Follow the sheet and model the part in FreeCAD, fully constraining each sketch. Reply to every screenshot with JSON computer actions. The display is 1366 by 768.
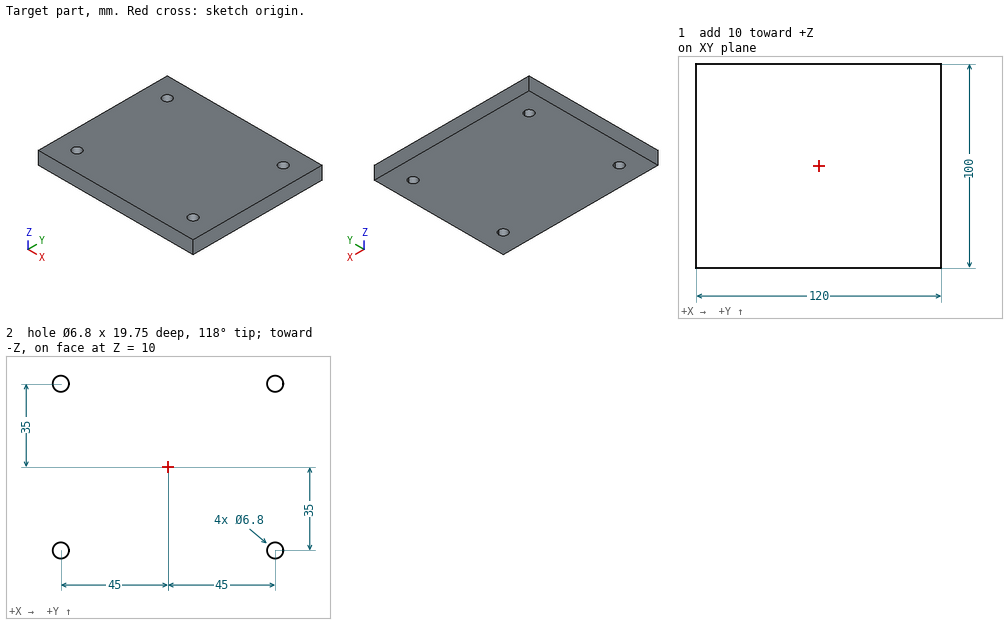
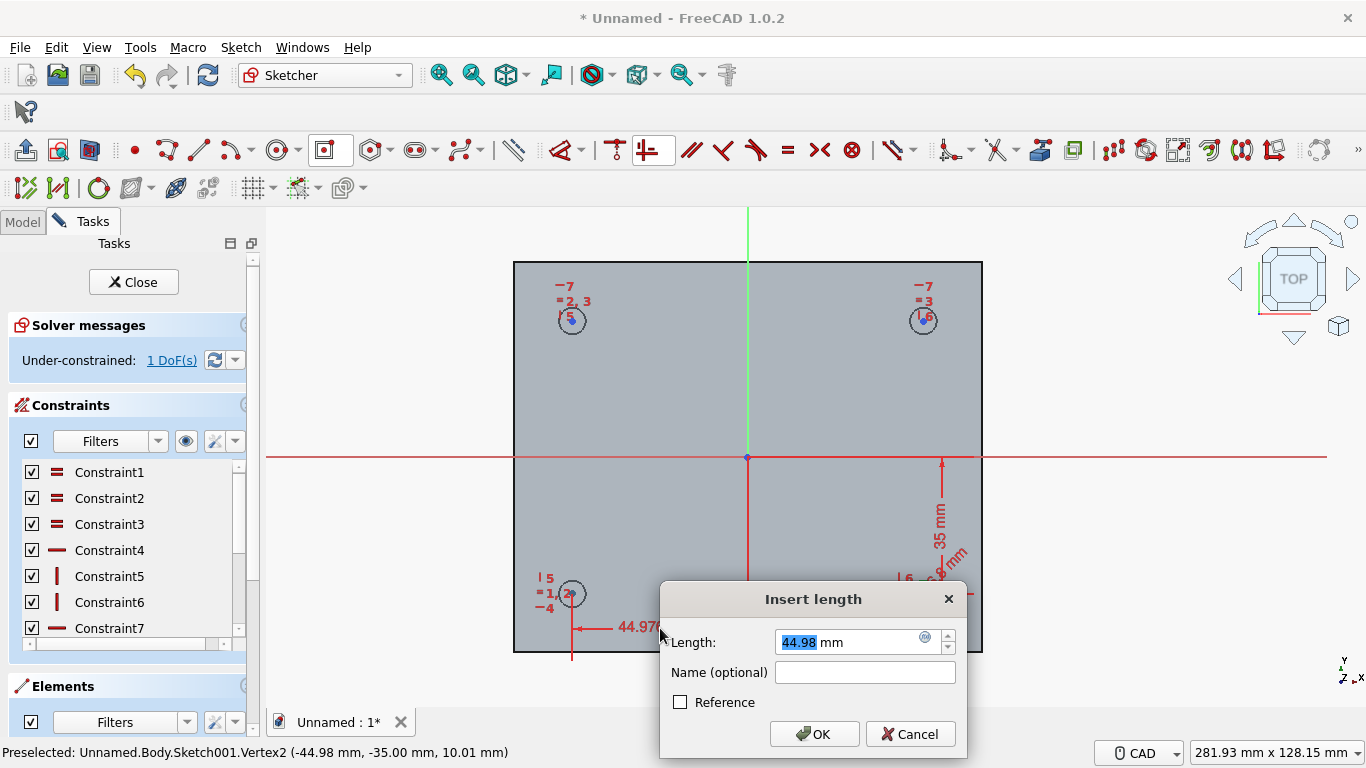
{"action": "type", "text": "45"}
{"action": "key", "text": "Return"}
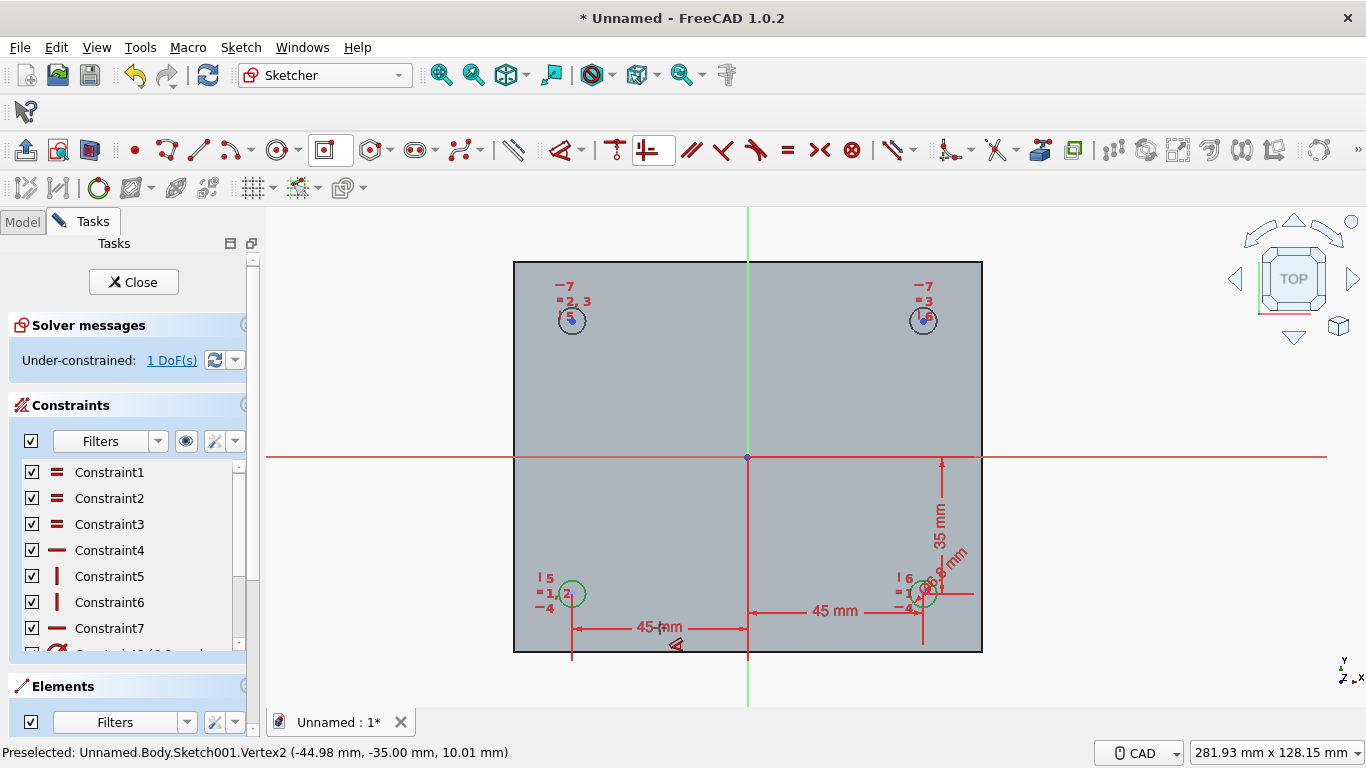
{"action": "left_click", "coordinate": [572, 321]}
{"action": "left_click", "coordinate": [538, 389]}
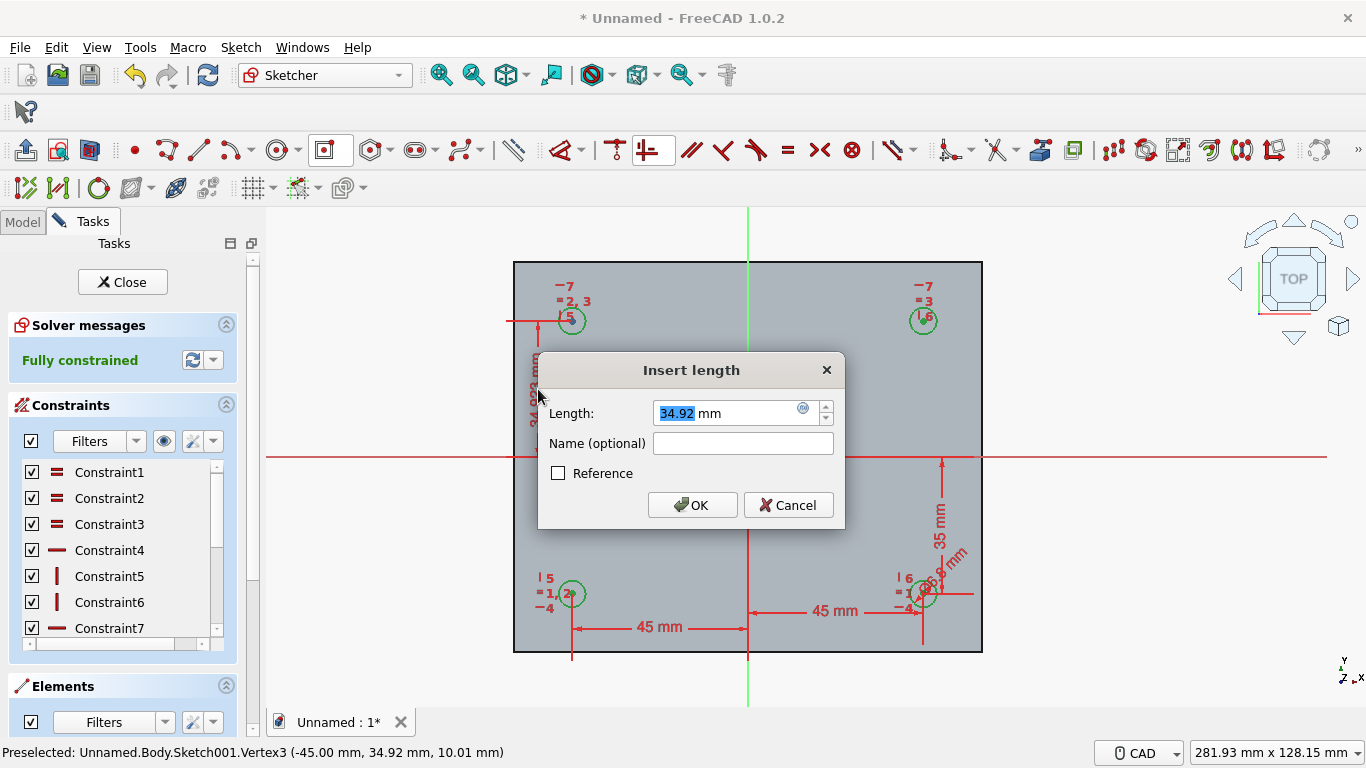
{"action": "type", "text": "35"}
{"action": "key", "text": "Return"}
{"action": "key", "text": "Escape"}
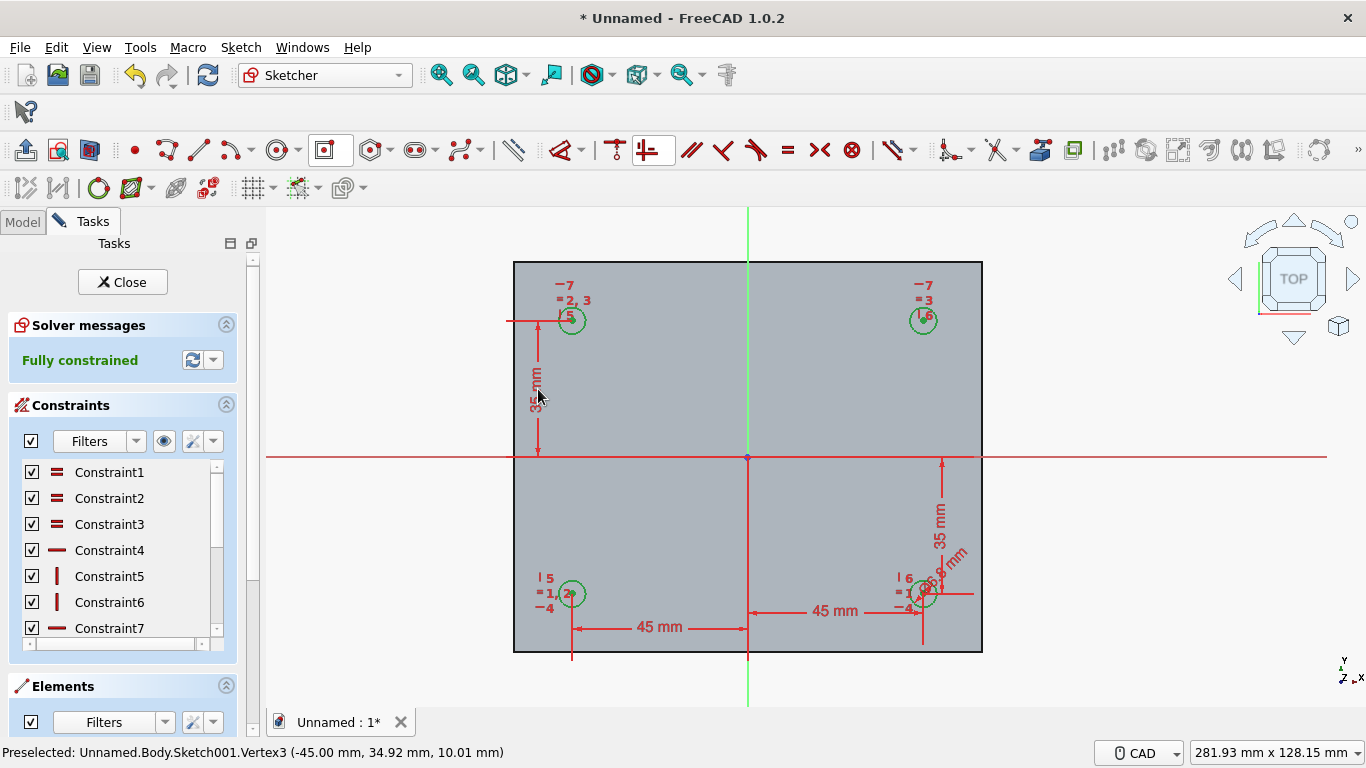
{"action": "left_click", "coordinate": [123, 282]}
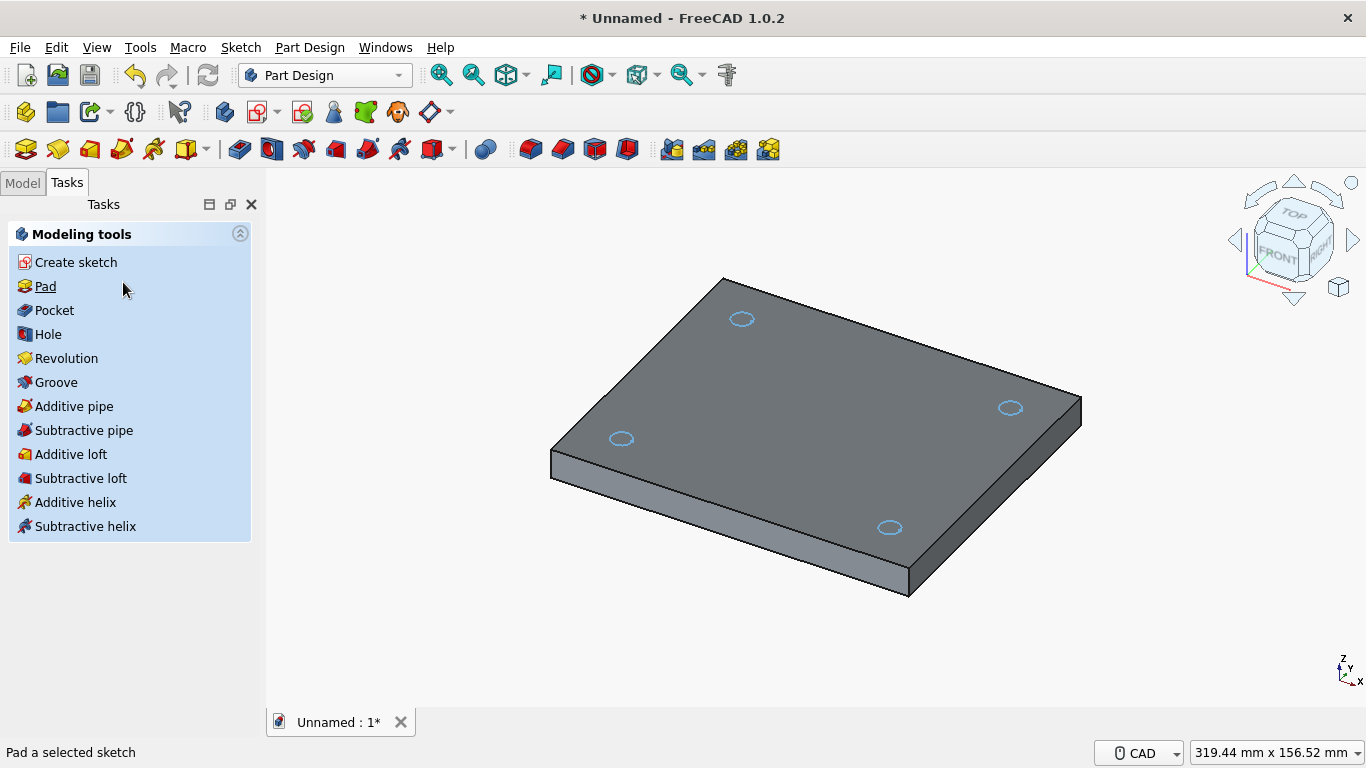
{"action": "left_click", "coordinate": [272, 150]}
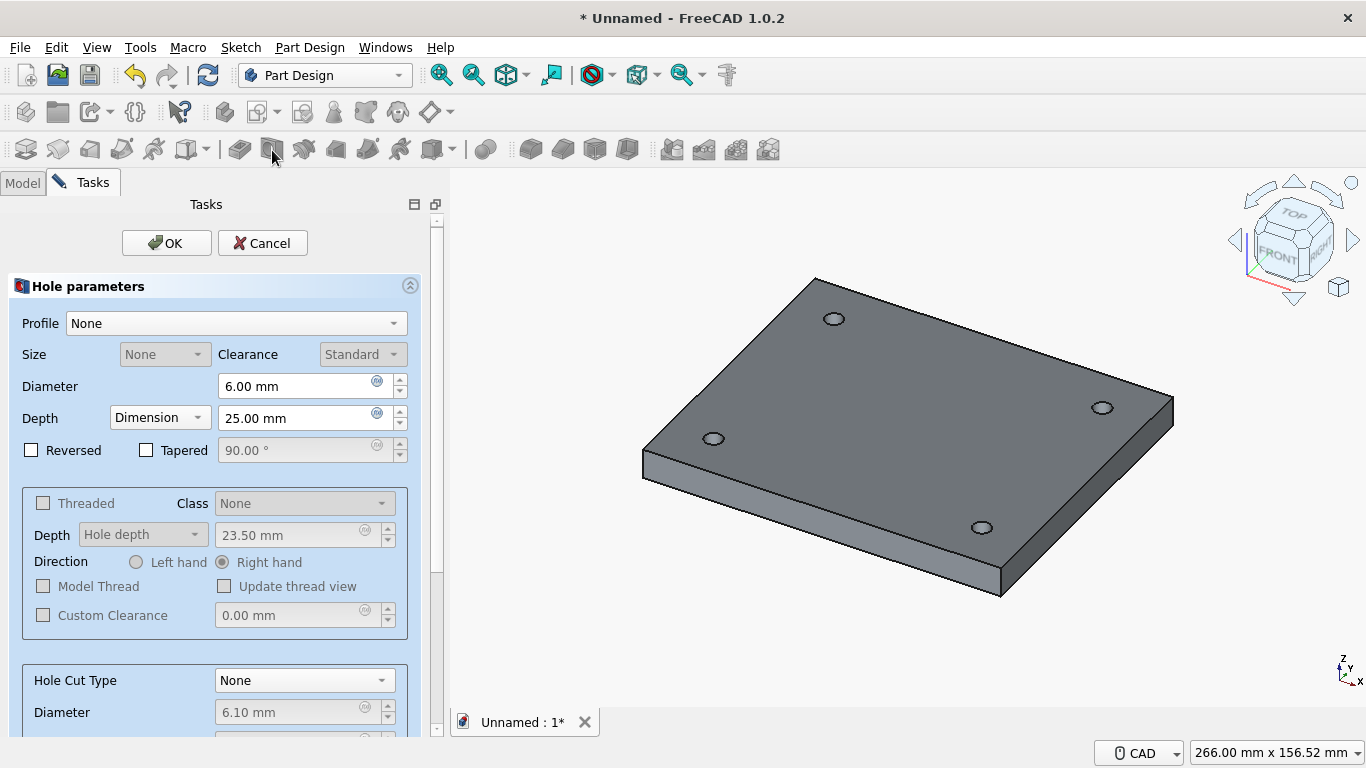
{"action": "triple_click", "coordinate": [305, 386]}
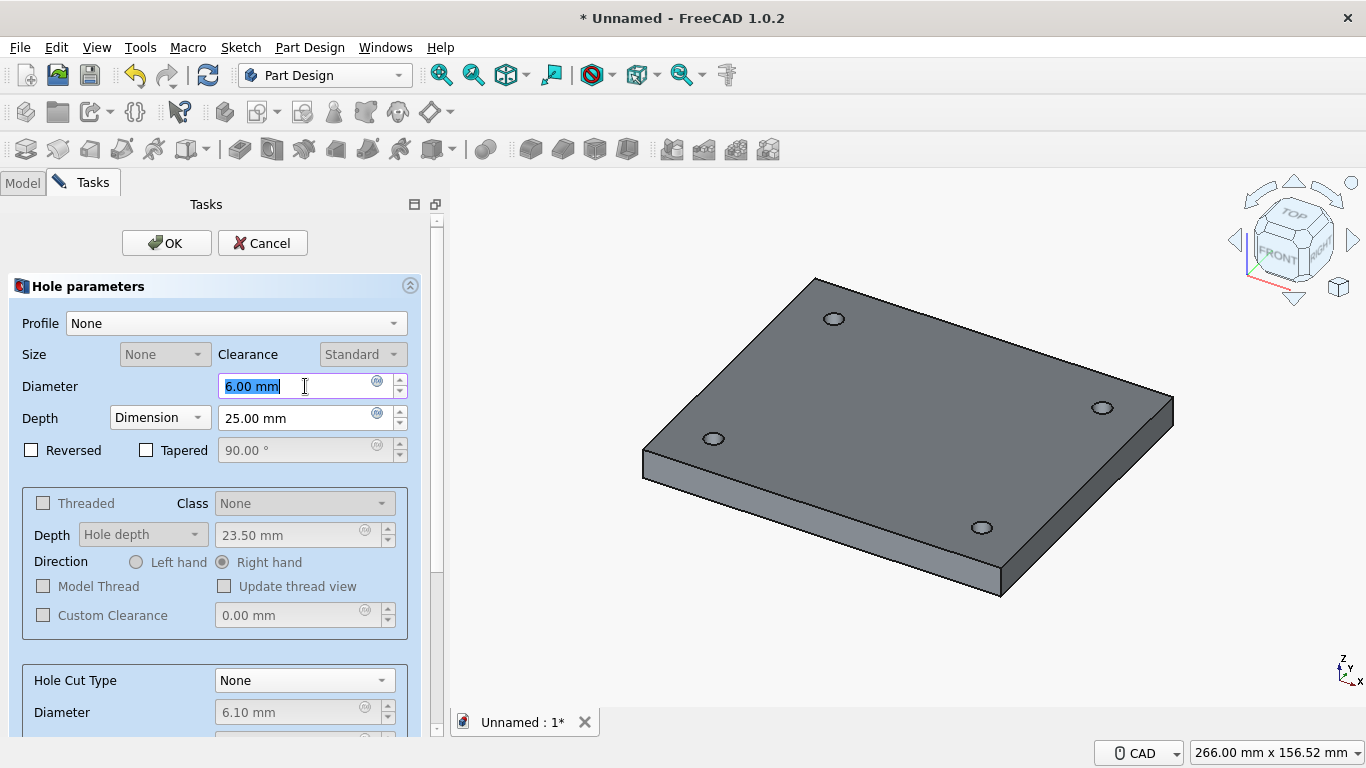
{"action": "type", "text": "6.8"}
{"action": "key", "text": "Tab"}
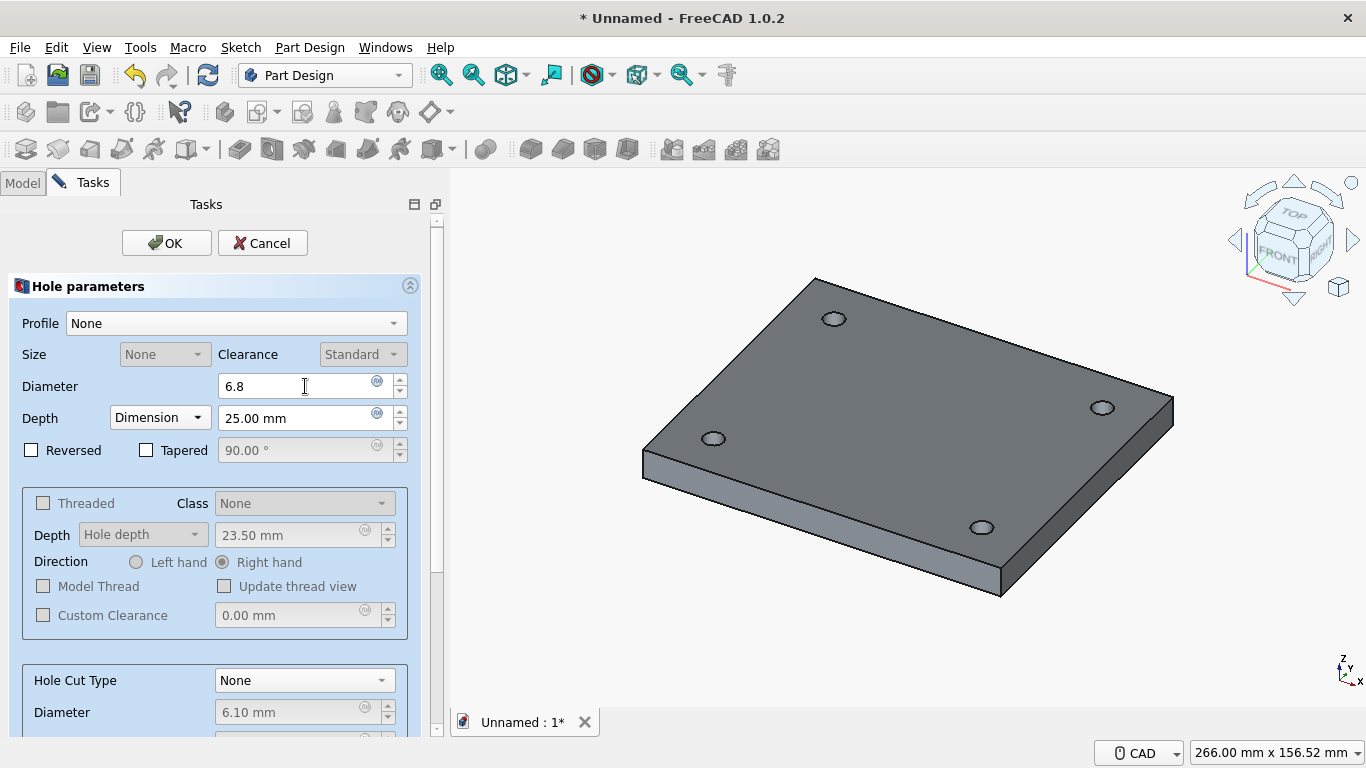
{"action": "triple_click", "coordinate": [305, 418]}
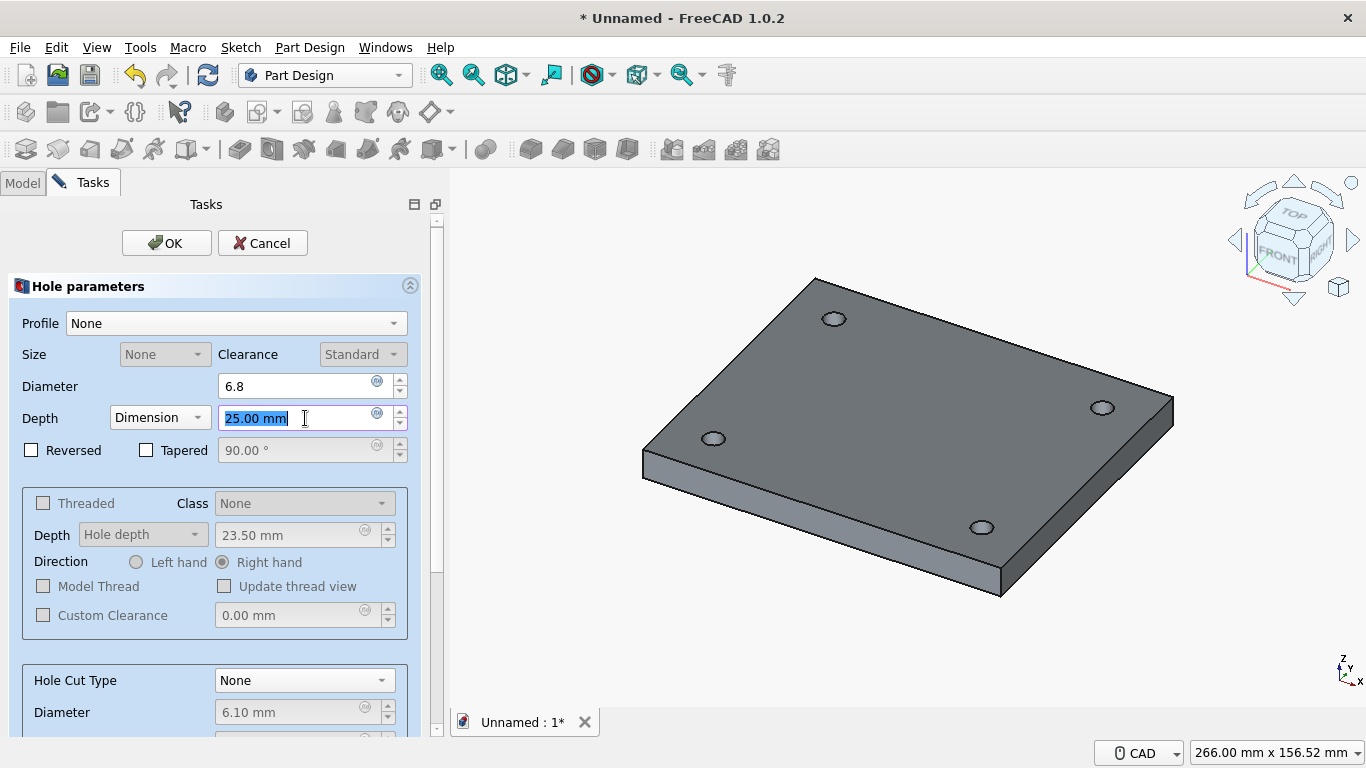
{"action": "type", "text": "19.75"}
{"action": "key", "text": "Tab"}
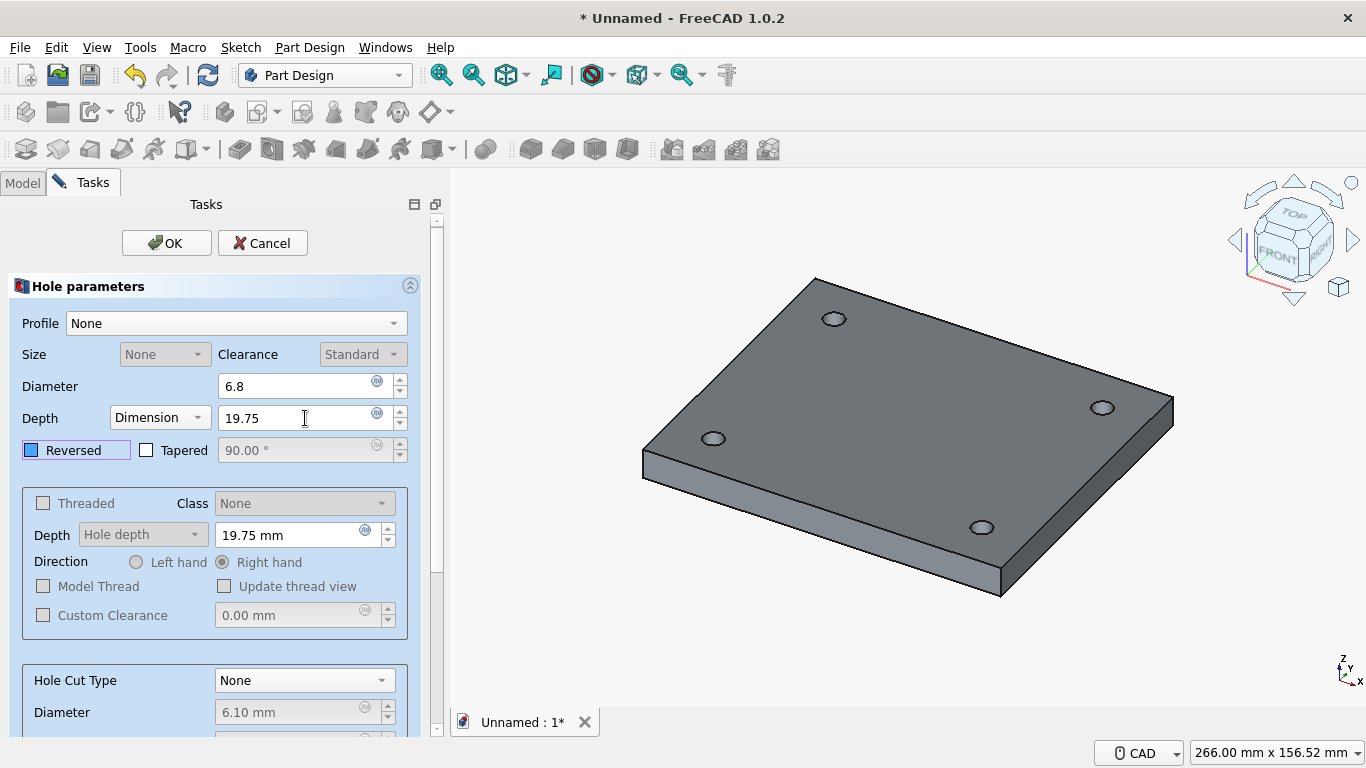
{"action": "left_click", "coordinate": [167, 243]}